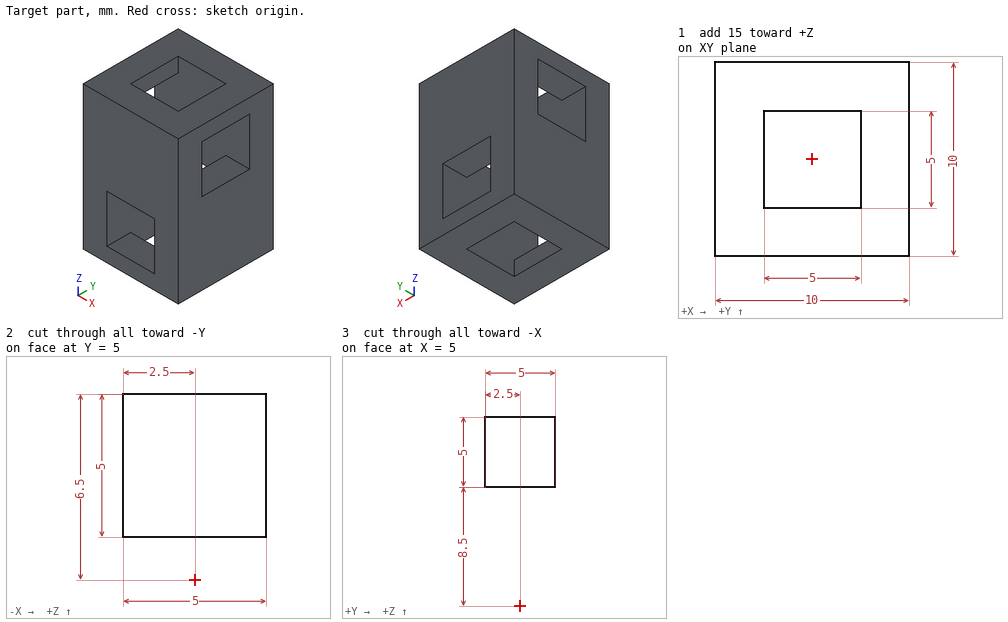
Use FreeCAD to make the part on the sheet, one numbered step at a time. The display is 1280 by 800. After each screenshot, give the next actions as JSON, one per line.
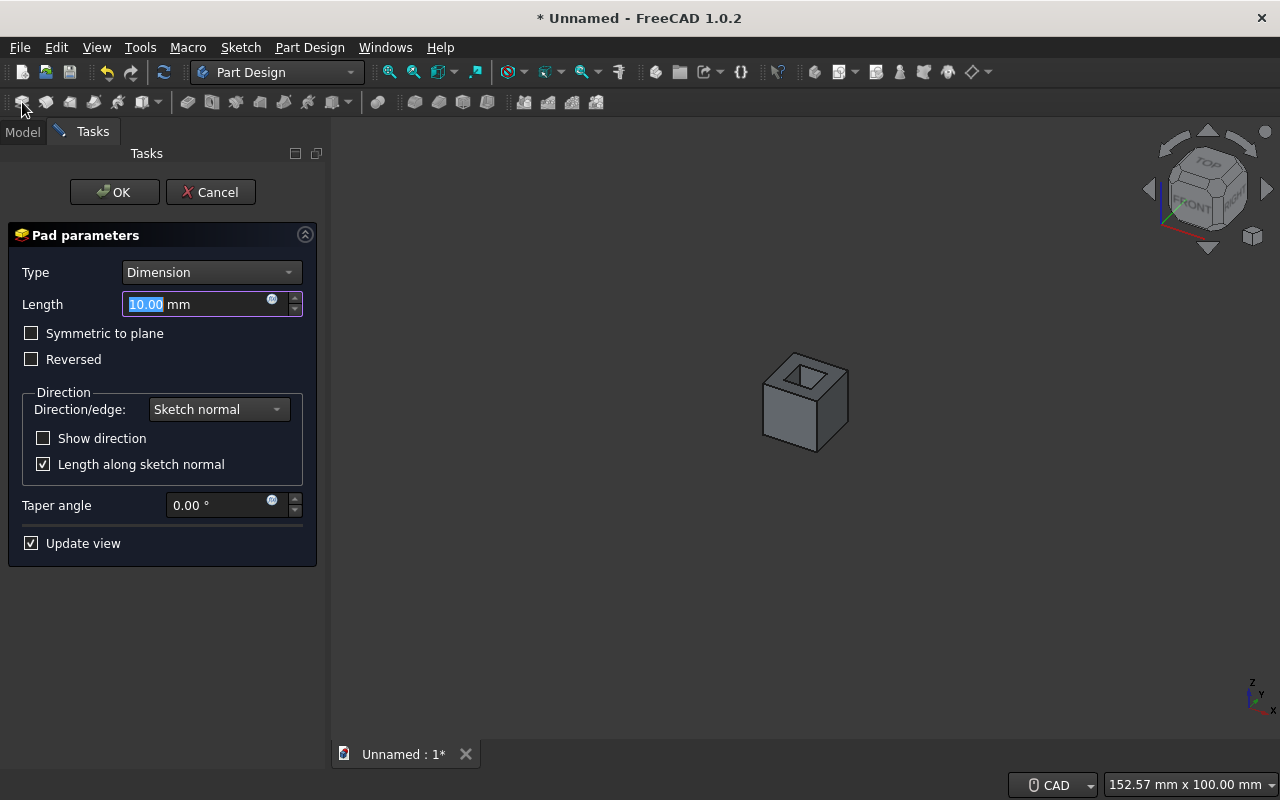
{"action": "type", "text": "15"}
{"action": "key", "text": "Tab"}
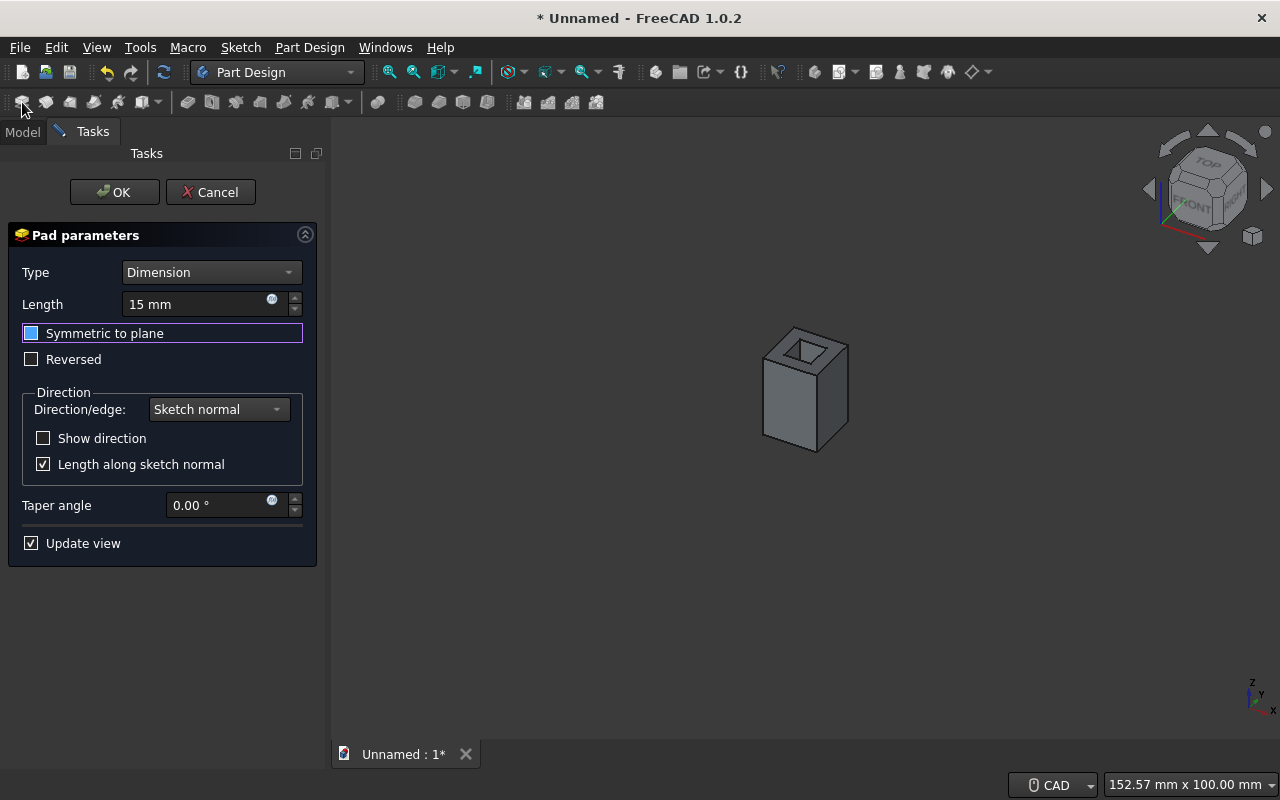
{"action": "left_click", "coordinate": [115, 192]}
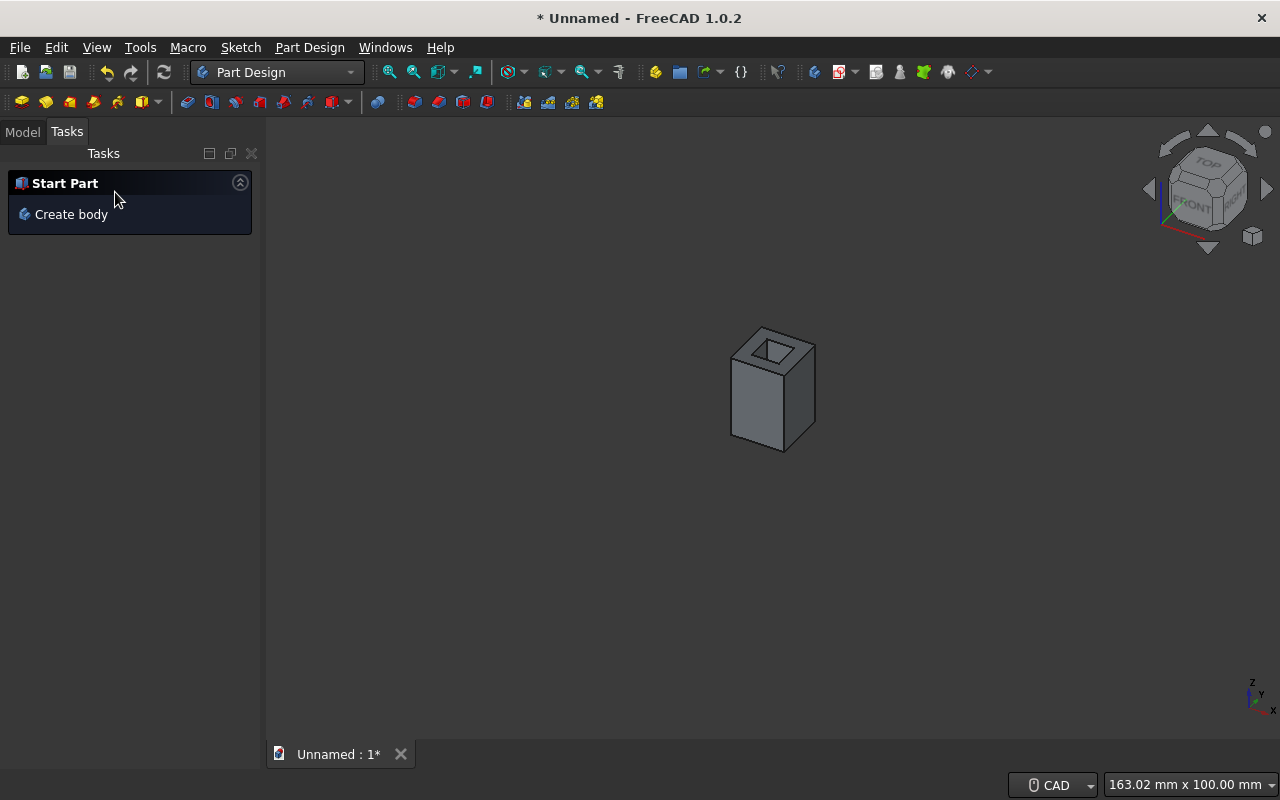
{"action": "left_click", "coordinate": [390, 72]}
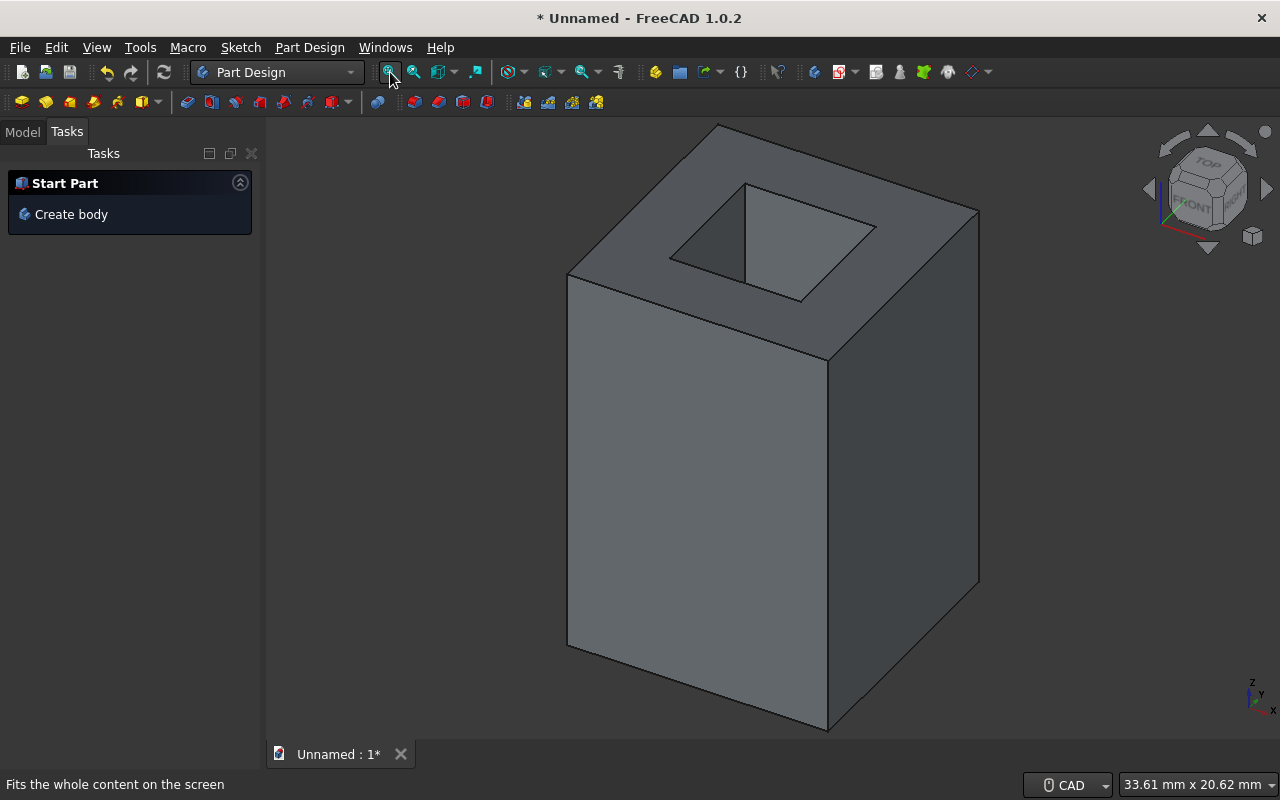
{"action": "key", "text": "4"}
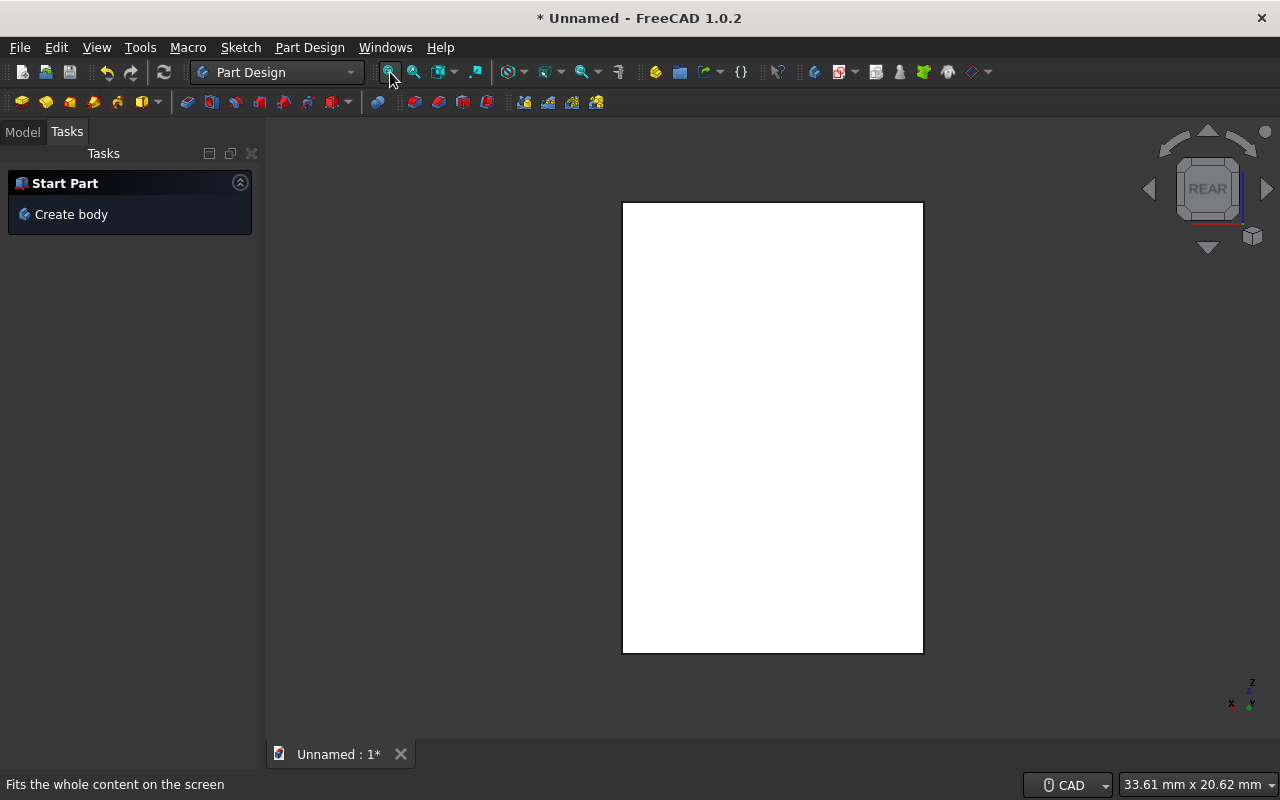
{"action": "left_click", "coordinate": [773, 362]}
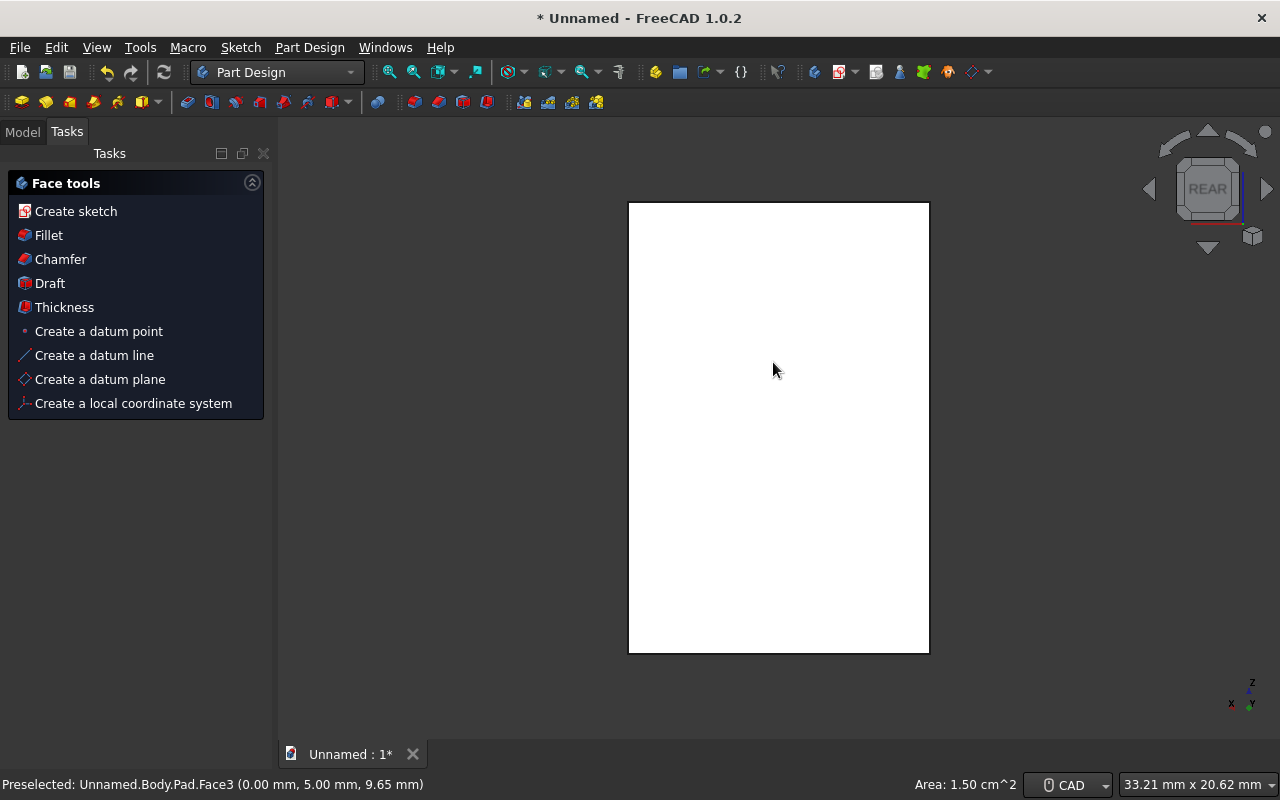
{"action": "left_click", "coordinate": [840, 72]}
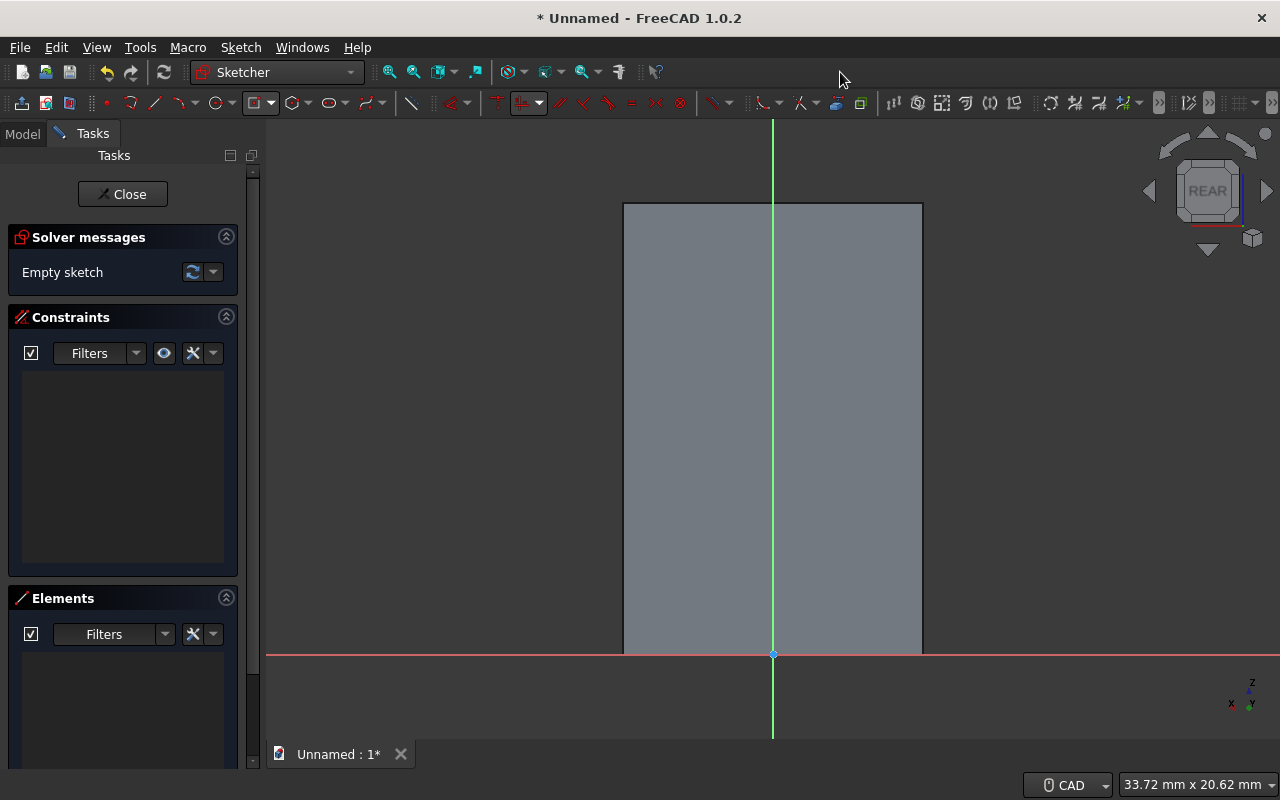
{"action": "scroll", "coordinate": [829, 661], "scroll_direction": "up", "scroll_amount": 4}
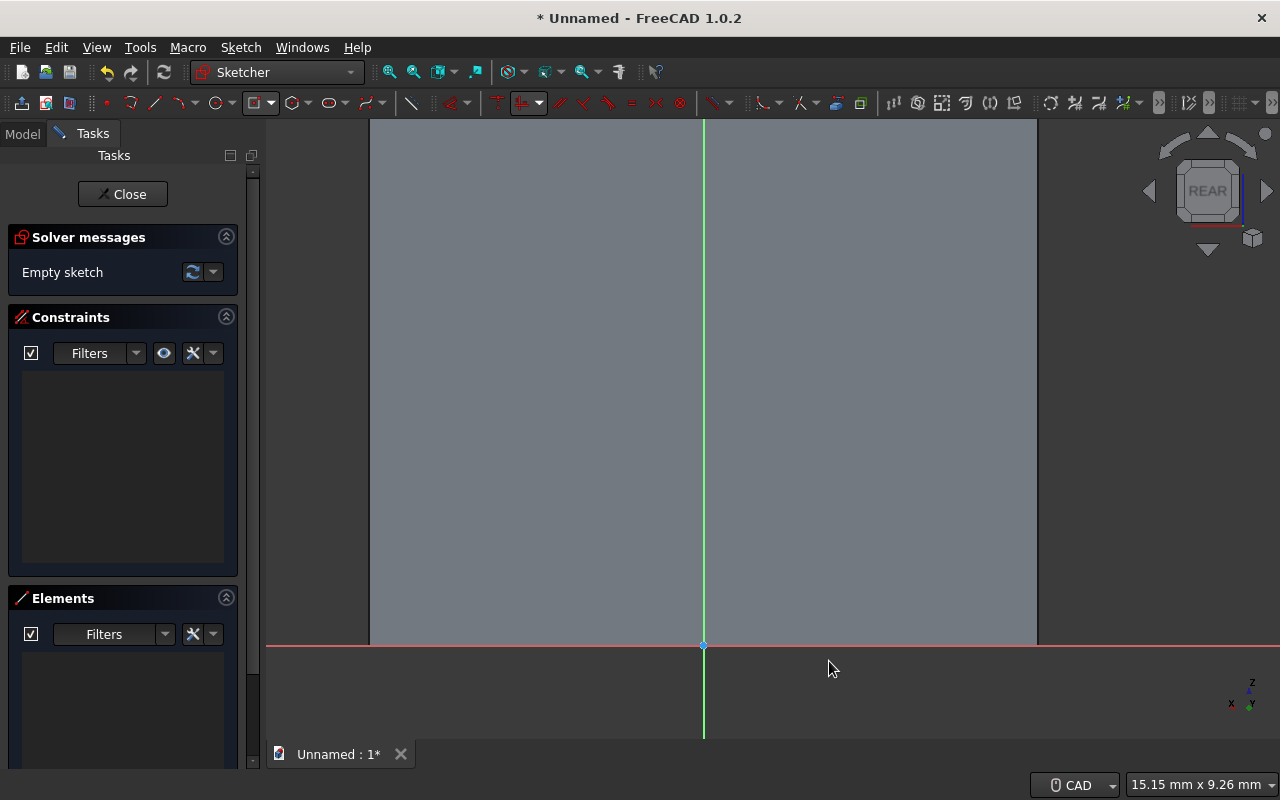
{"action": "key", "text": "g r"}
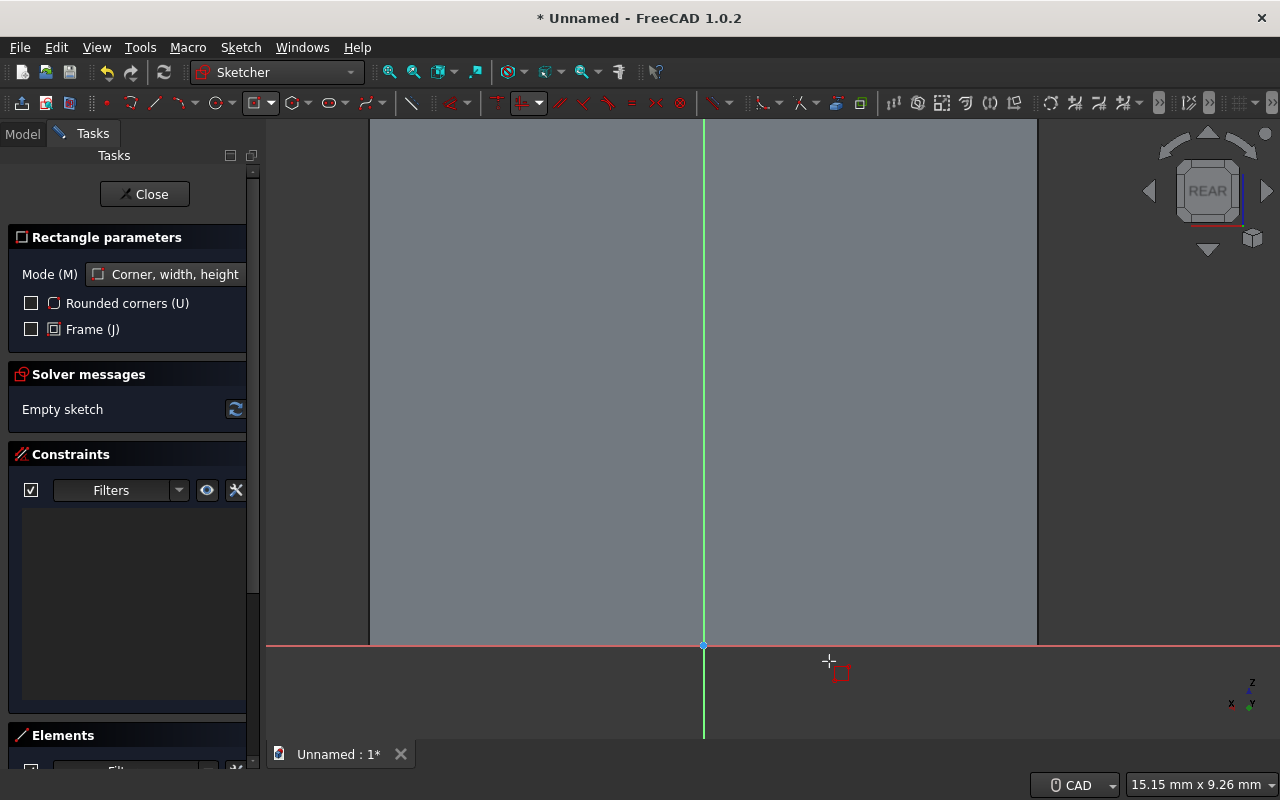
{"action": "left_click", "coordinate": [536, 211]}
{"action": "left_click", "coordinate": [871, 545]}
{"action": "key", "text": "Escape"}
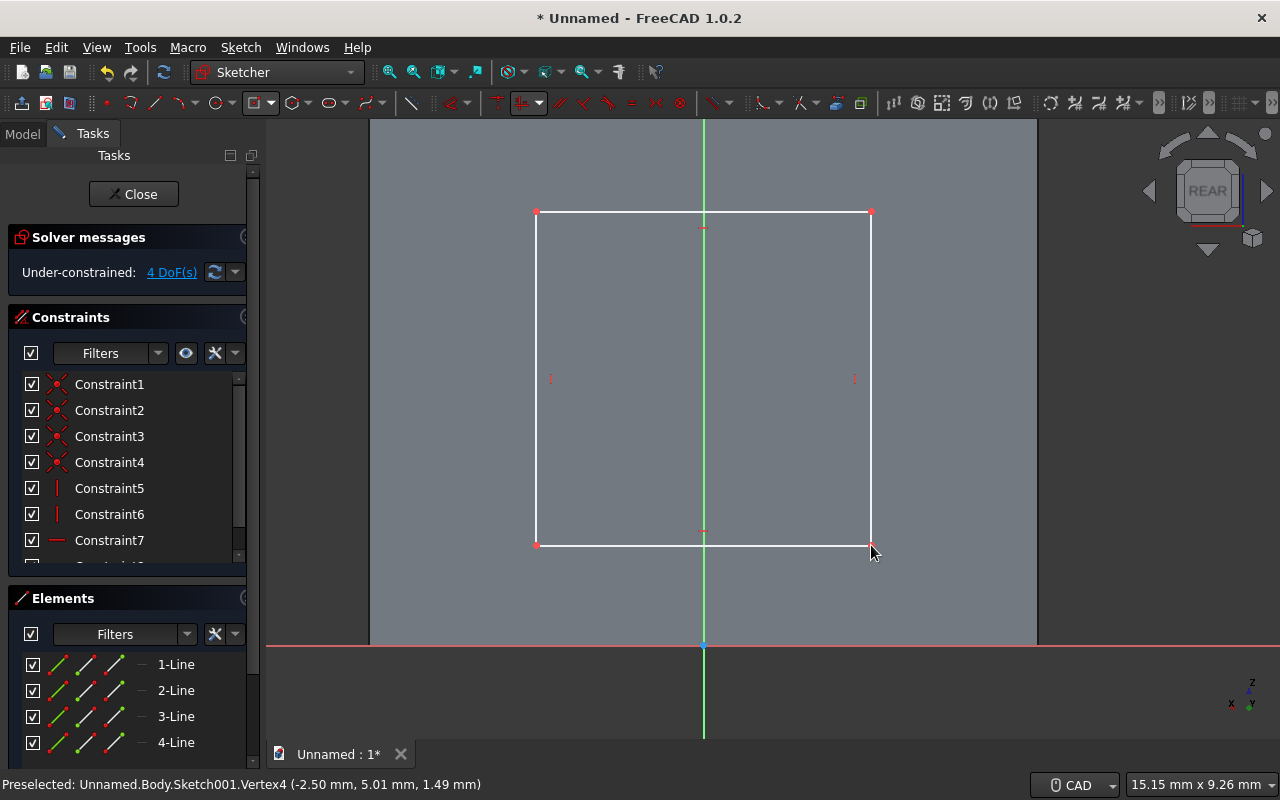
{"action": "left_click", "coordinate": [450, 104]}